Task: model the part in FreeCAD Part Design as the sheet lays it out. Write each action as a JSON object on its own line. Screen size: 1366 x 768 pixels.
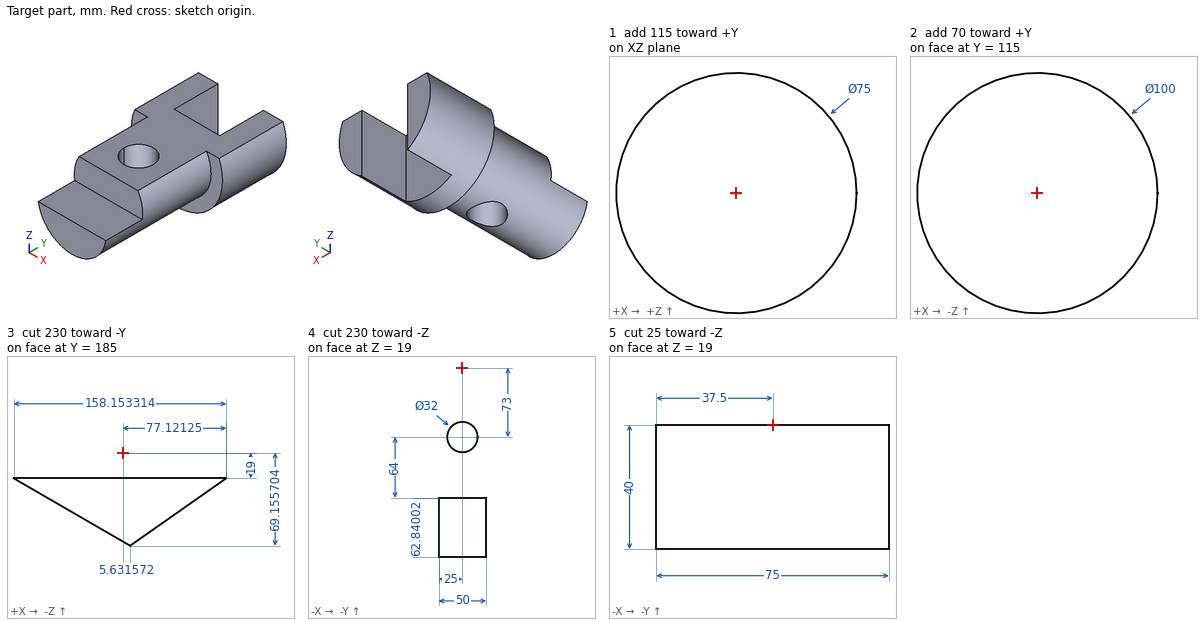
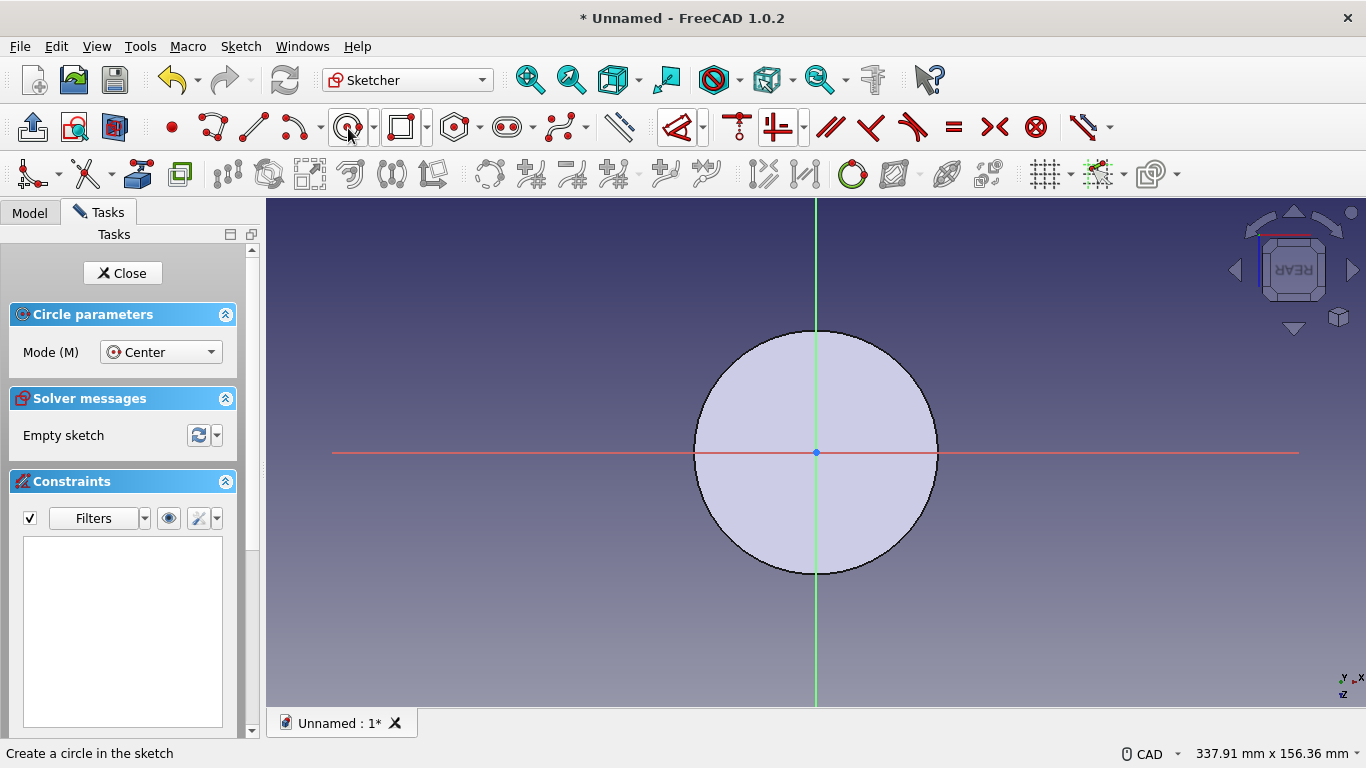
{"action": "left_click", "coordinate": [816, 452]}
{"action": "left_click", "coordinate": [931, 337]}
{"action": "key", "text": "Escape"}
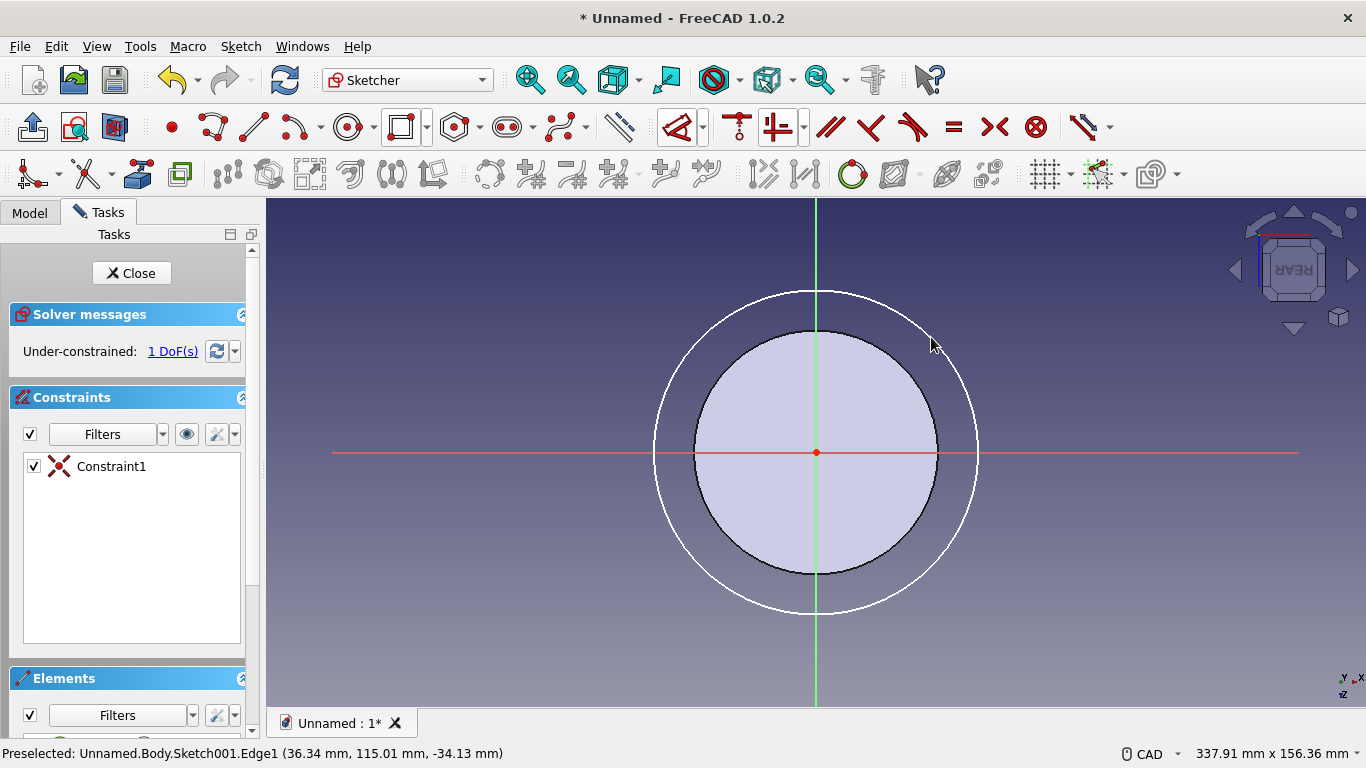
{"action": "left_click", "coordinate": [930, 337]}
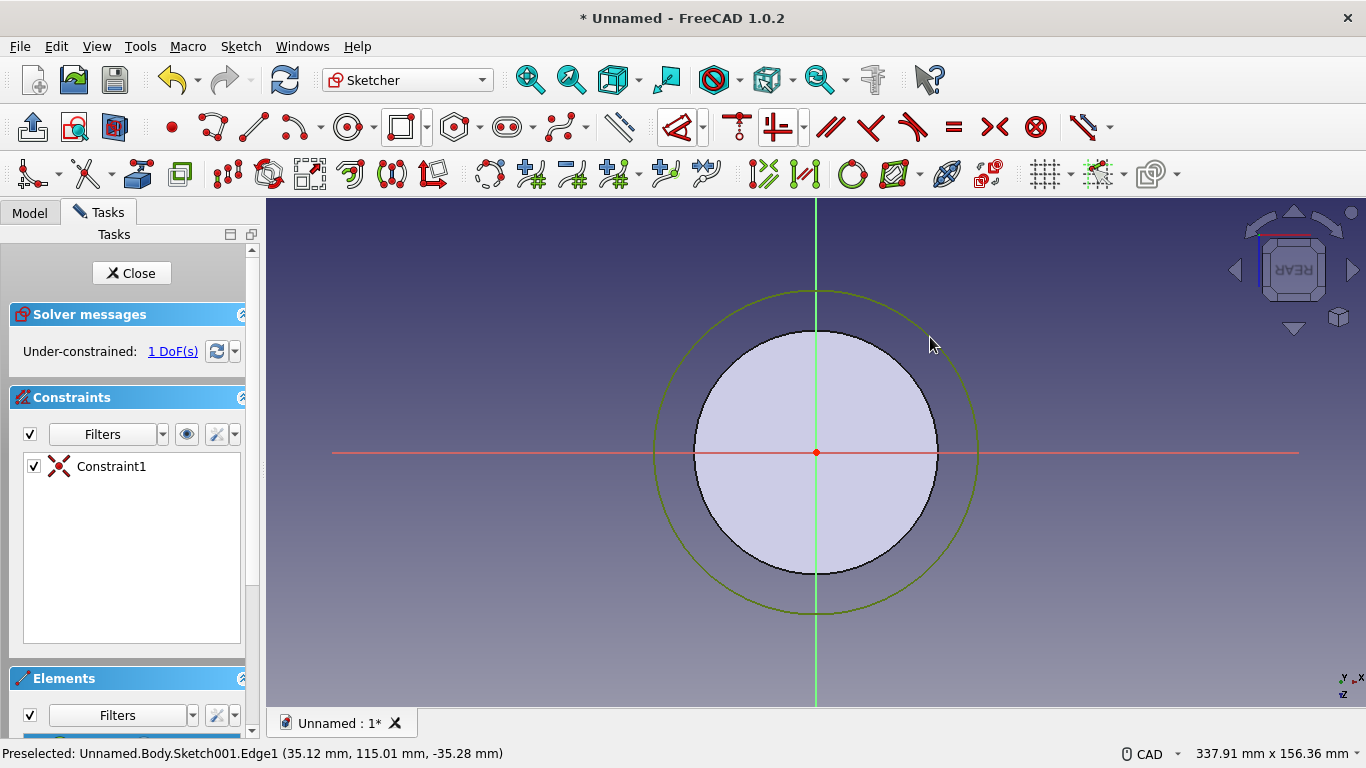
{"action": "left_click", "coordinate": [702, 128]}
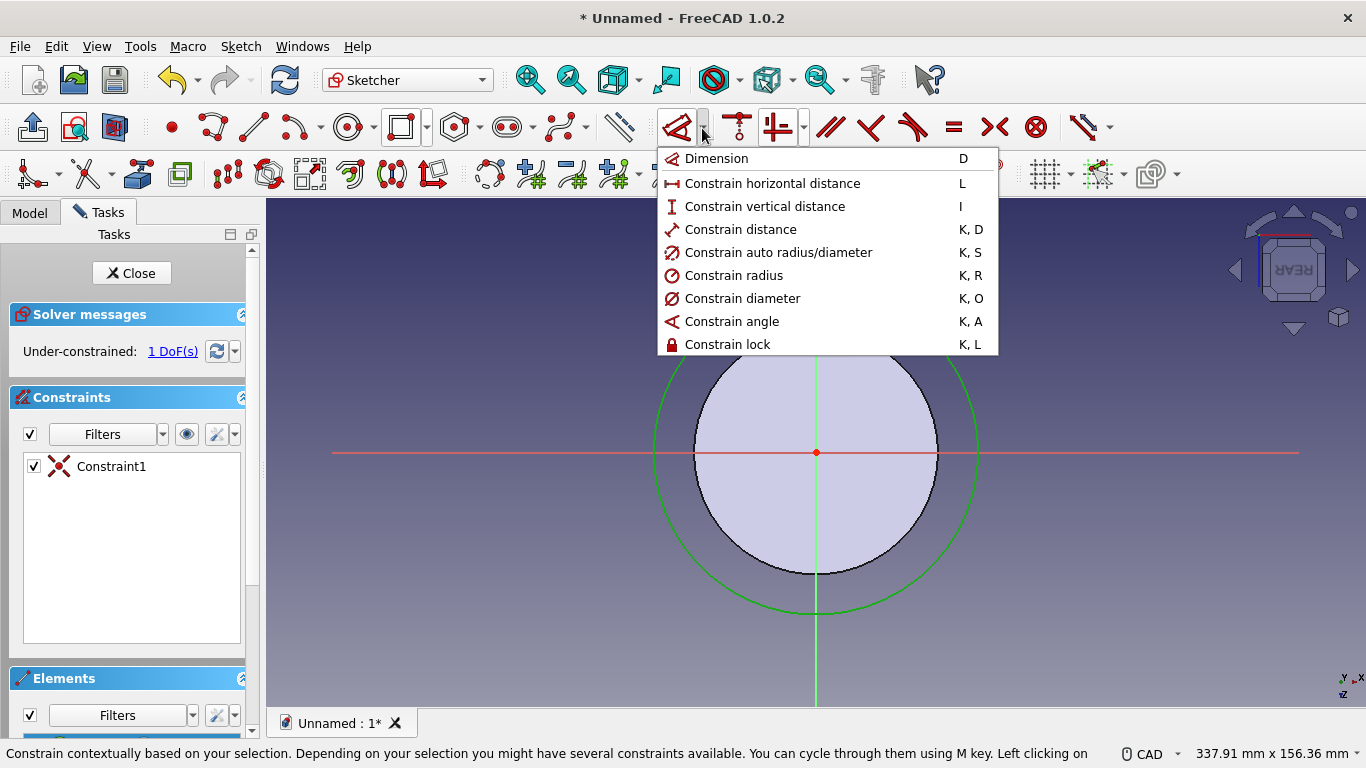
{"action": "left_click", "coordinate": [828, 298]}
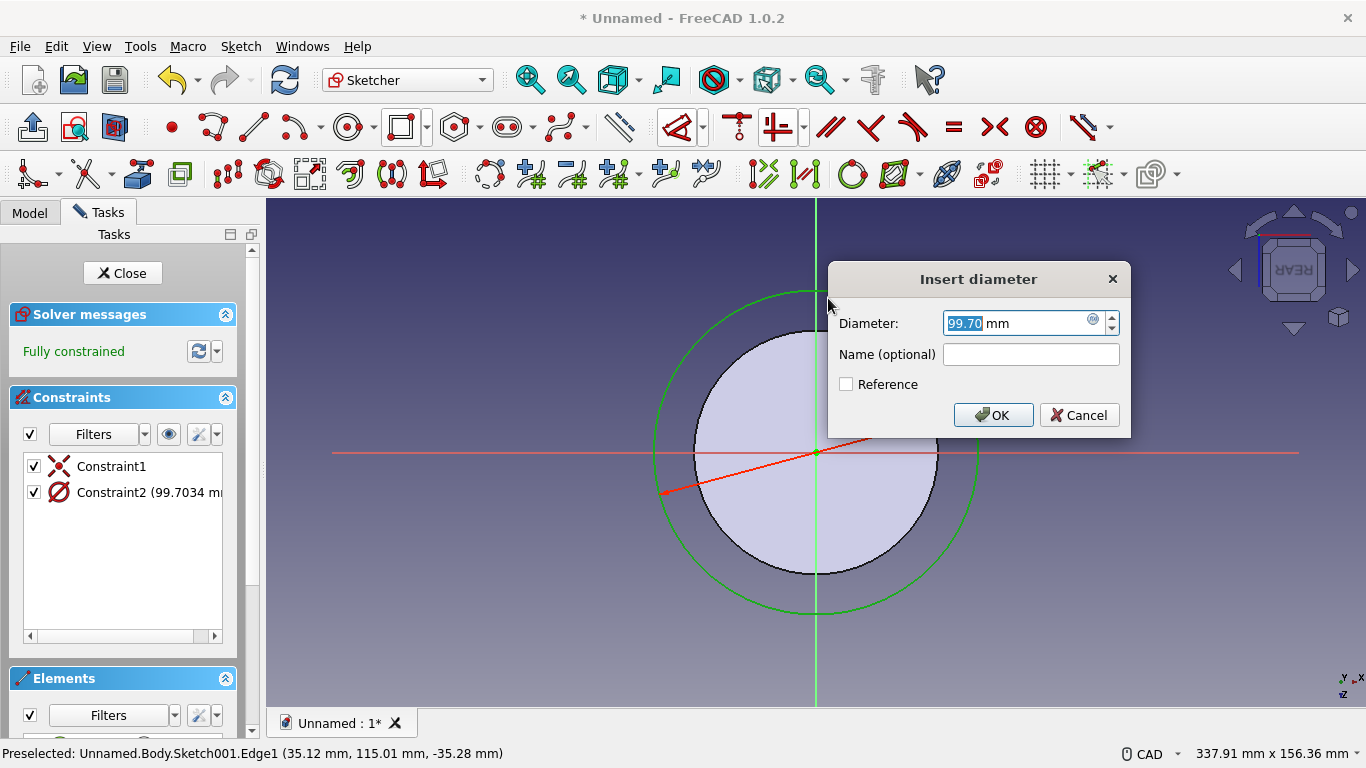
{"action": "type", "text": "100"}
{"action": "key", "text": "Return"}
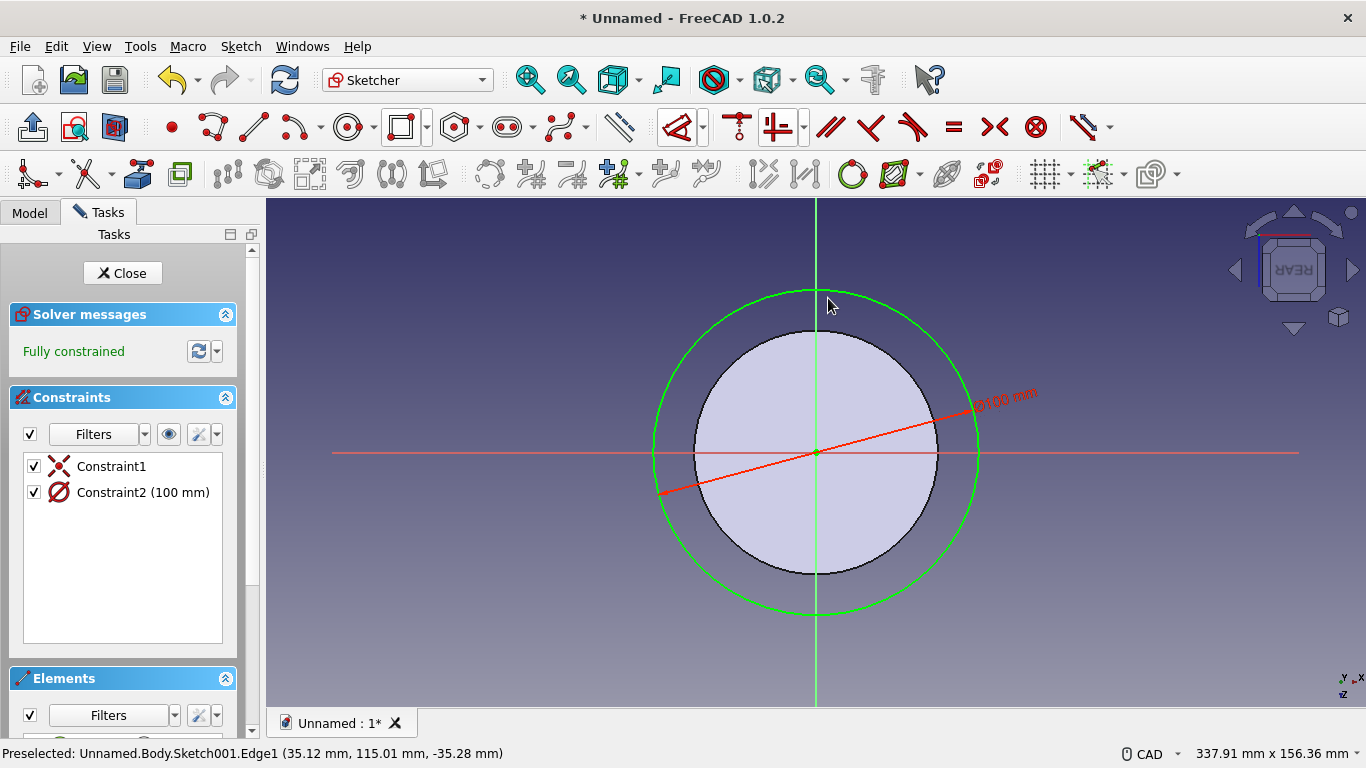
{"action": "left_click", "coordinate": [123, 273]}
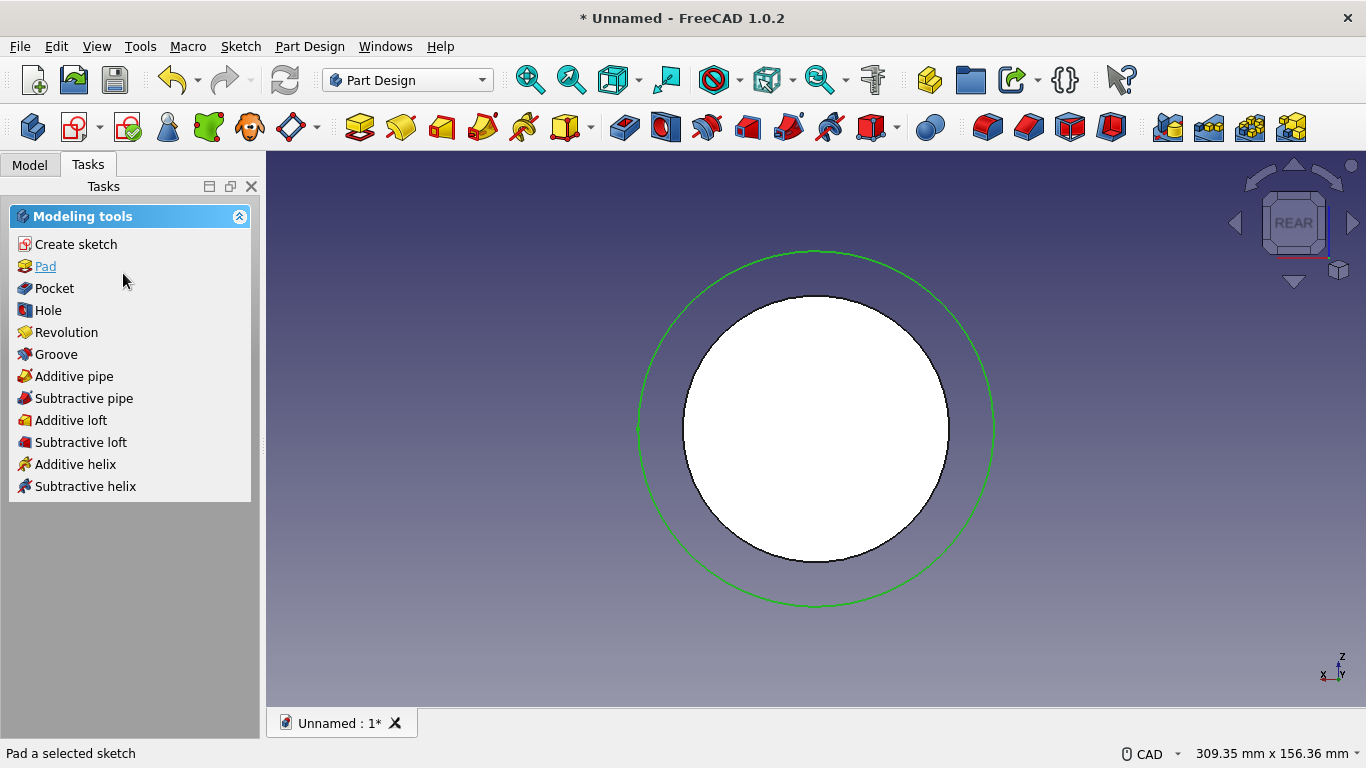
{"action": "left_click", "coordinate": [360, 128]}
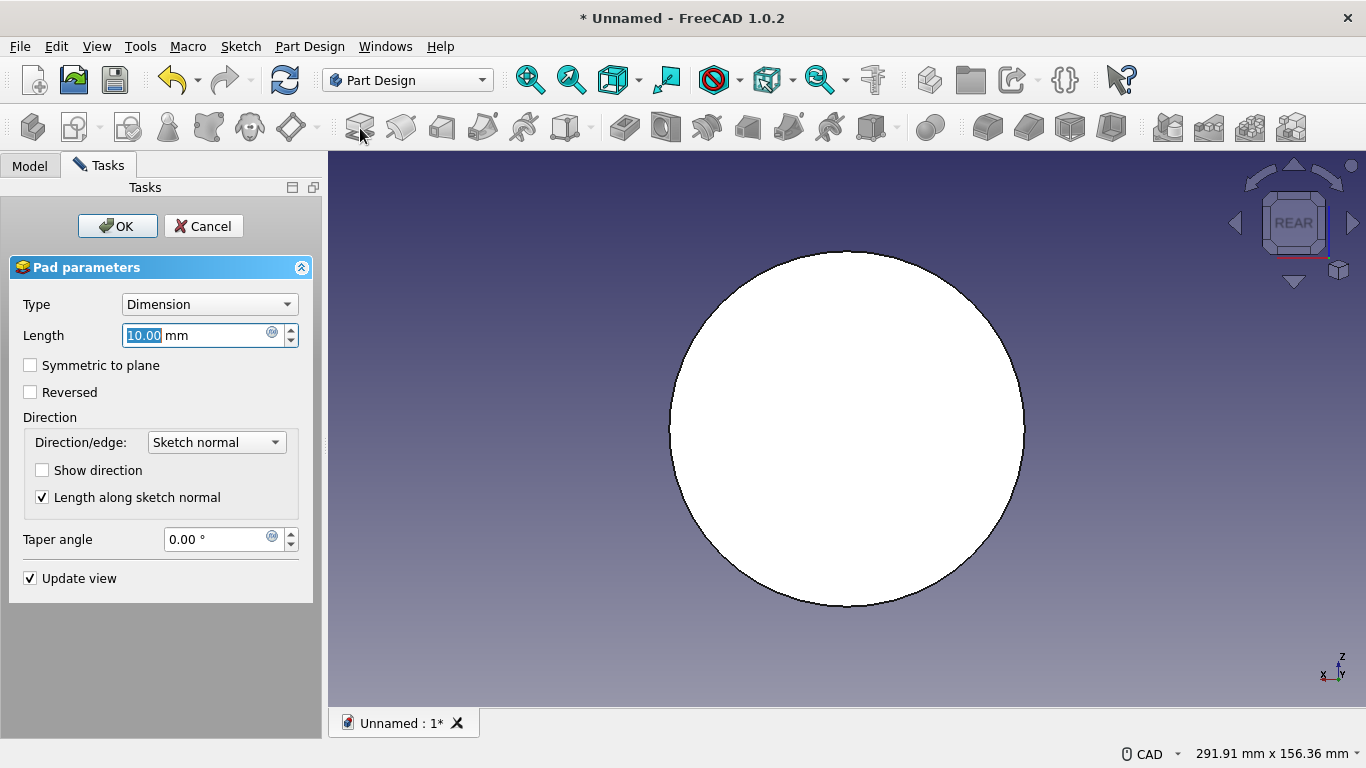
{"action": "type", "text": "70"}
{"action": "key", "text": "Tab"}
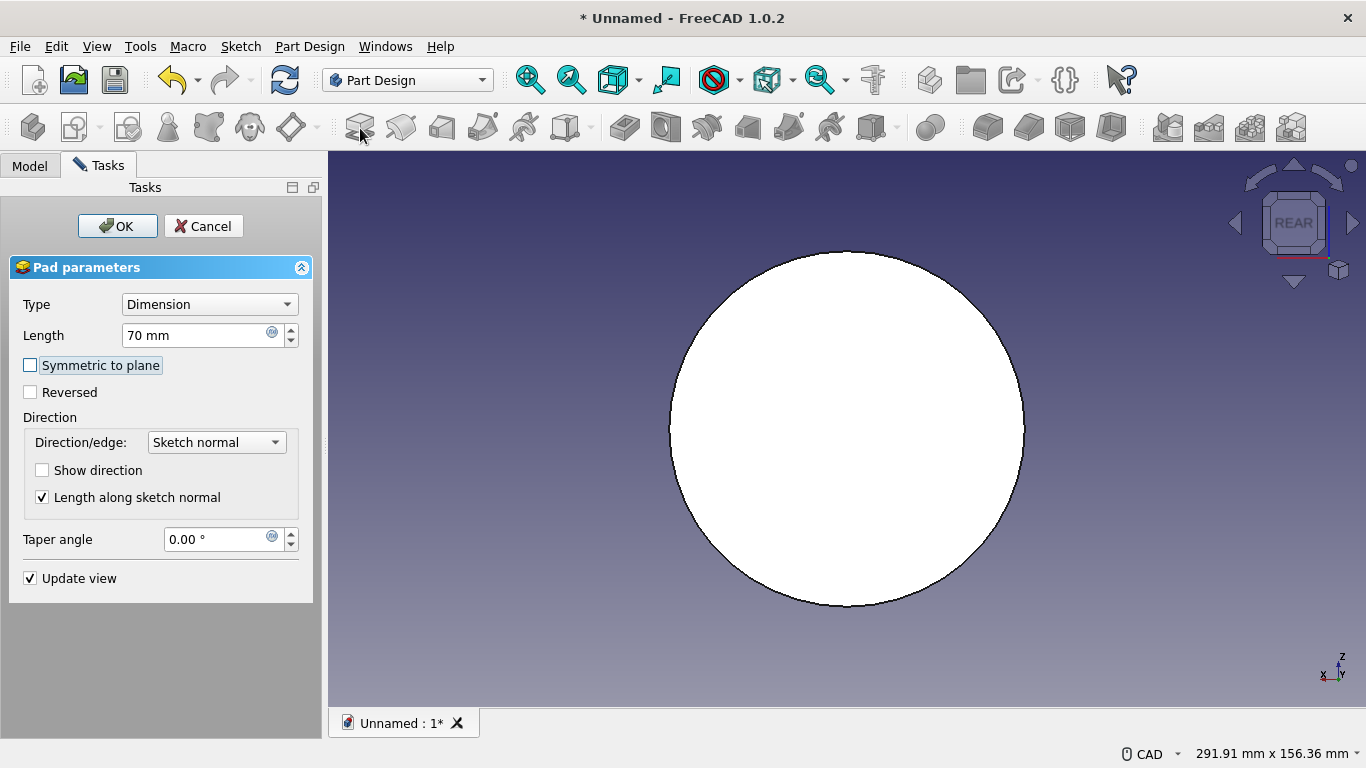
{"action": "left_click", "coordinate": [118, 226]}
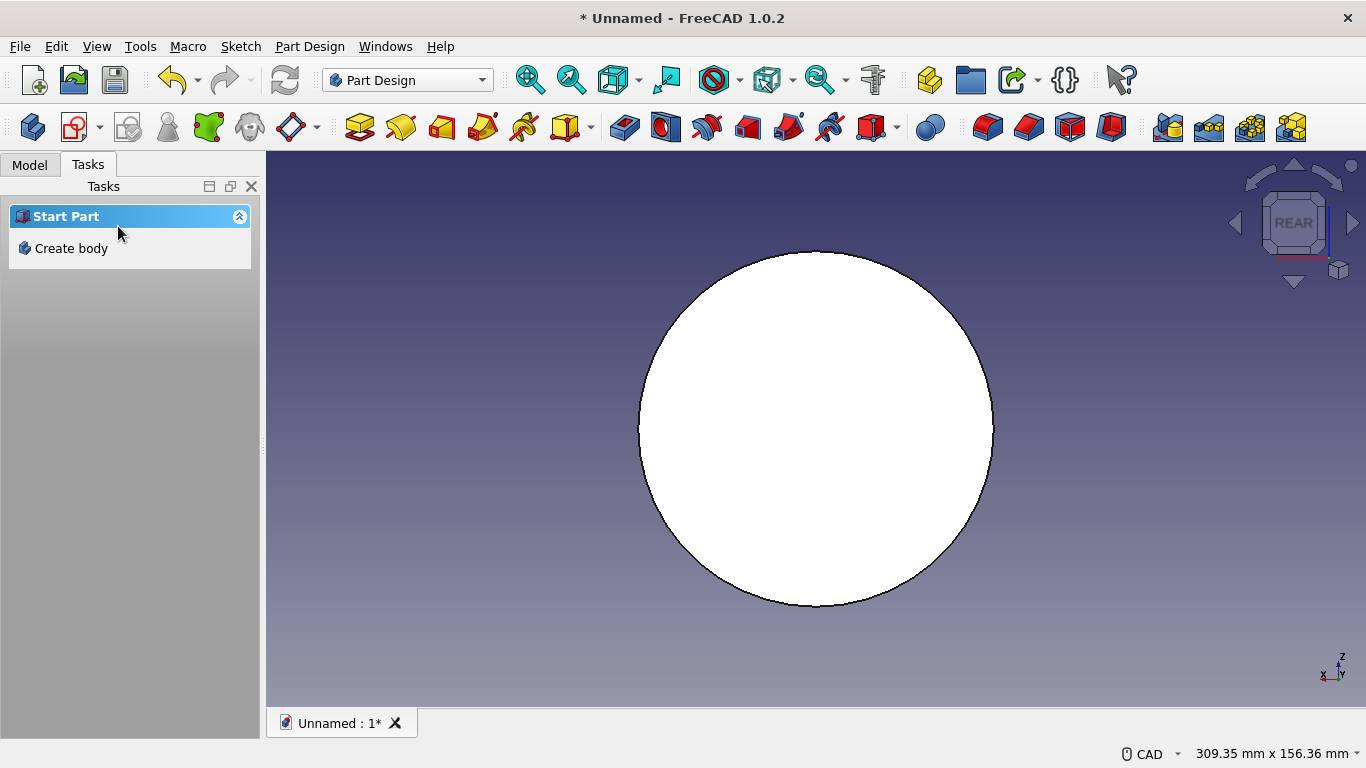
{"action": "left_click", "coordinate": [816, 428]}